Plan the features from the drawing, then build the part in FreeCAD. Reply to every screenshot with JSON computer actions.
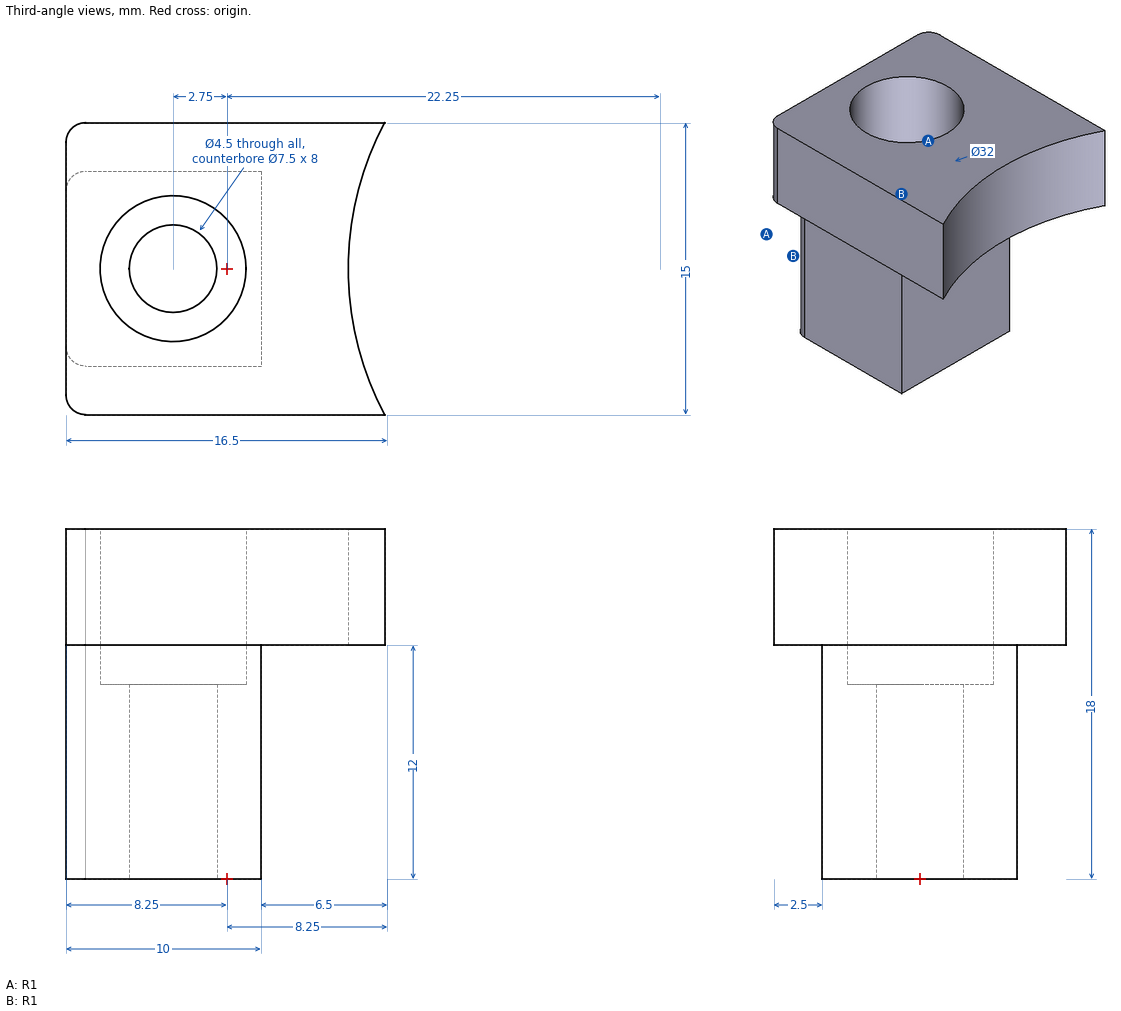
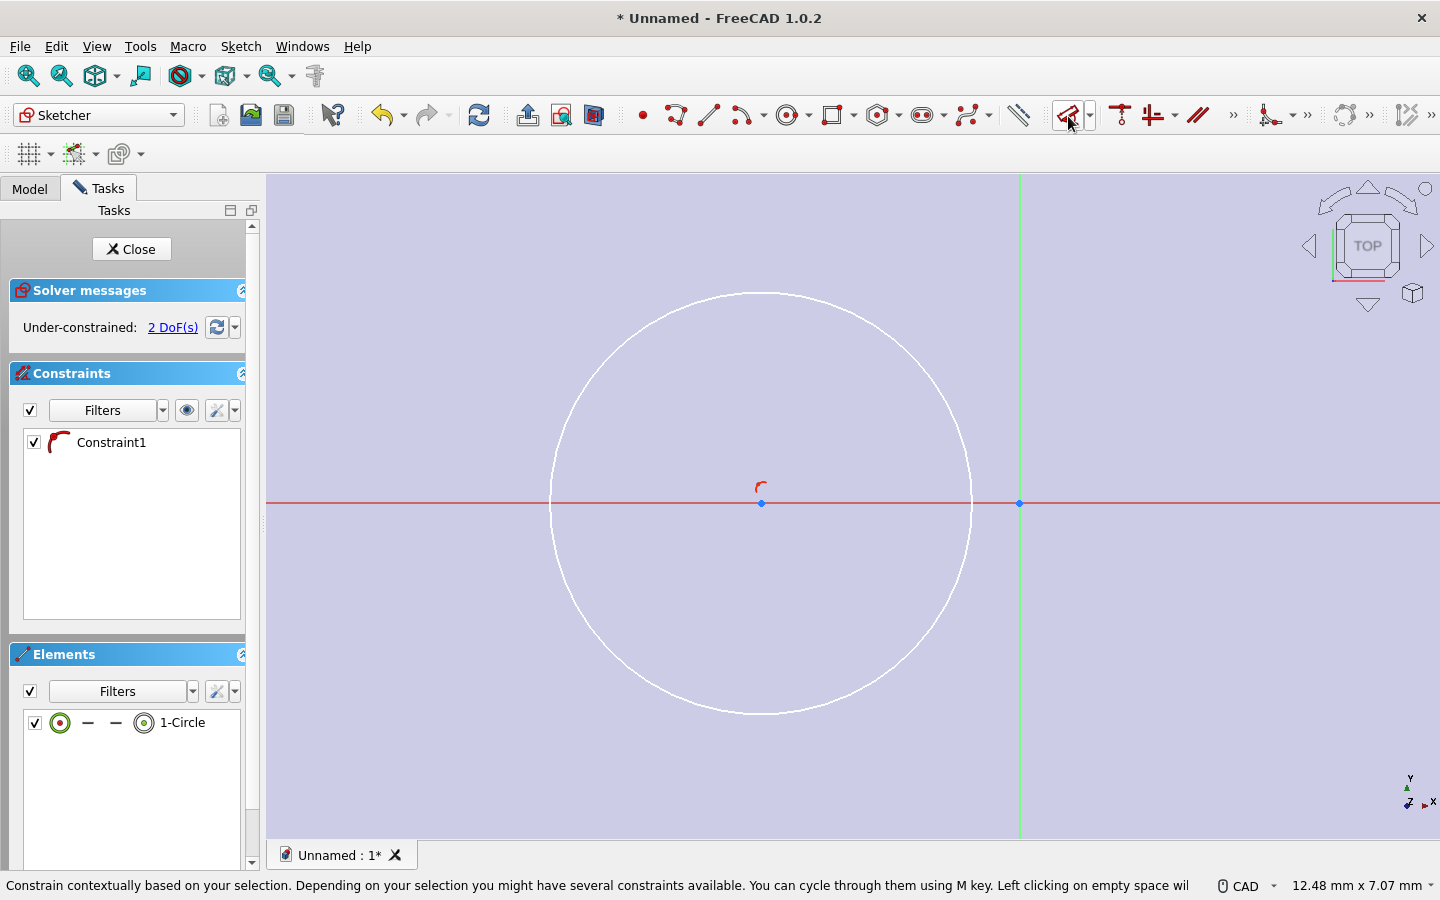
{"action": "left_click", "coordinate": [910, 354]}
{"action": "left_click", "coordinate": [933, 331]}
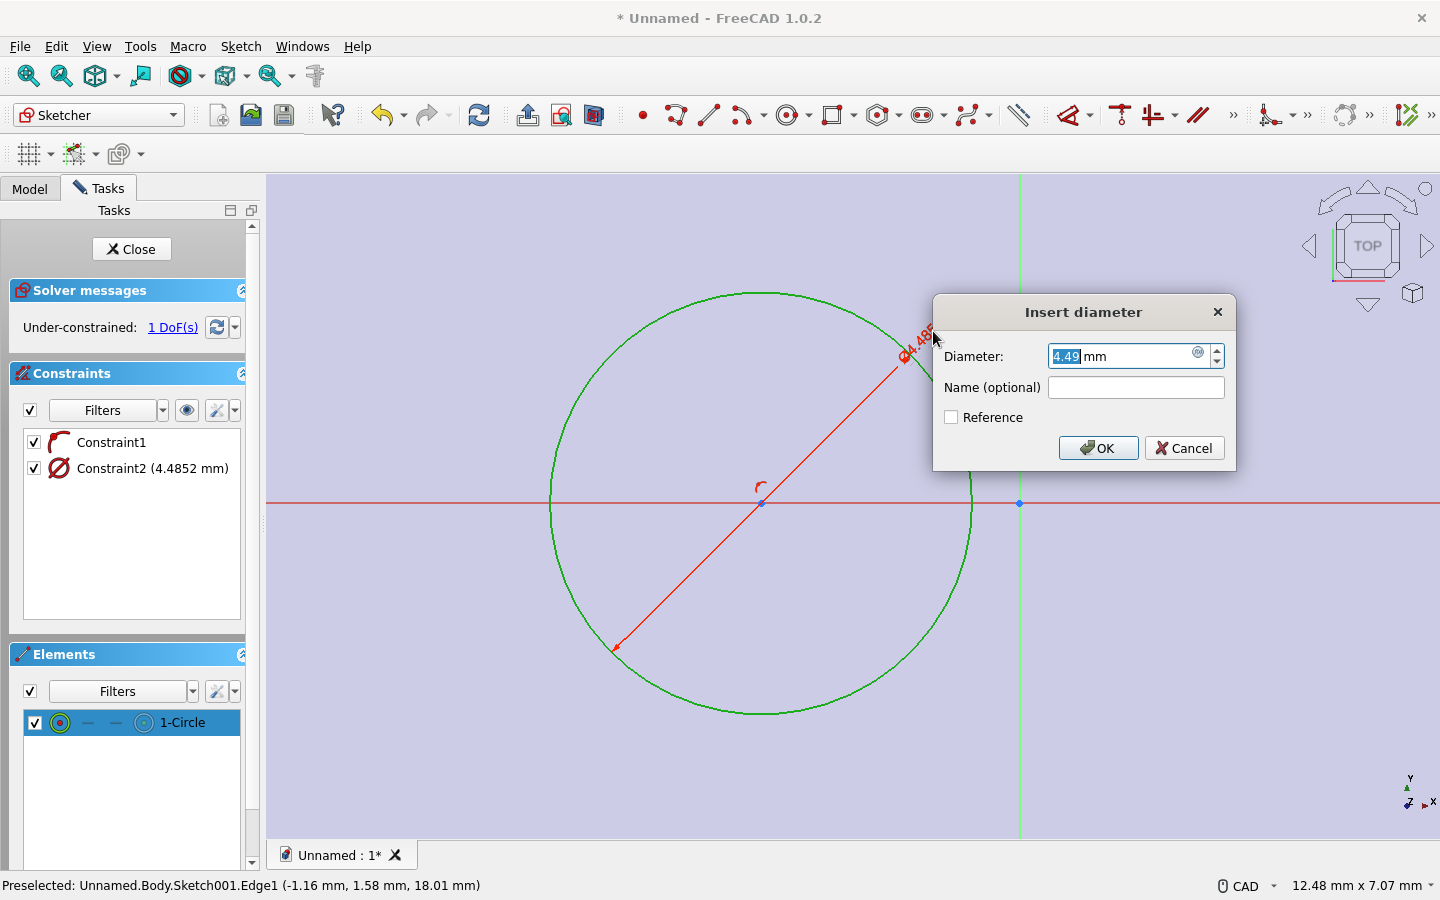
{"action": "type", "text": "4.5"}
{"action": "key", "text": "Return"}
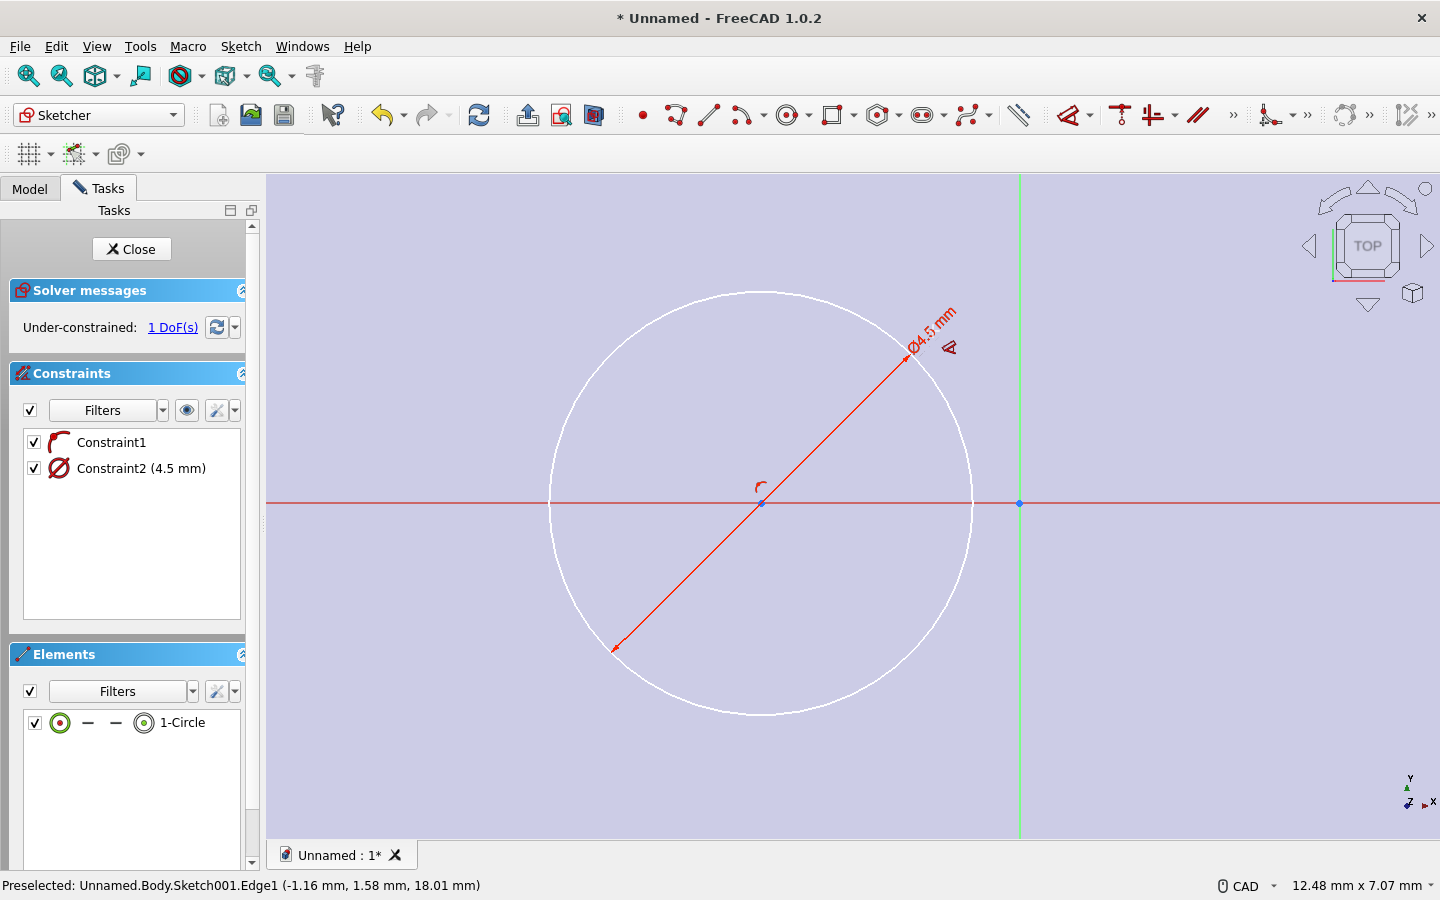
{"action": "left_click", "coordinate": [761, 503]}
{"action": "left_click", "coordinate": [890, 537]}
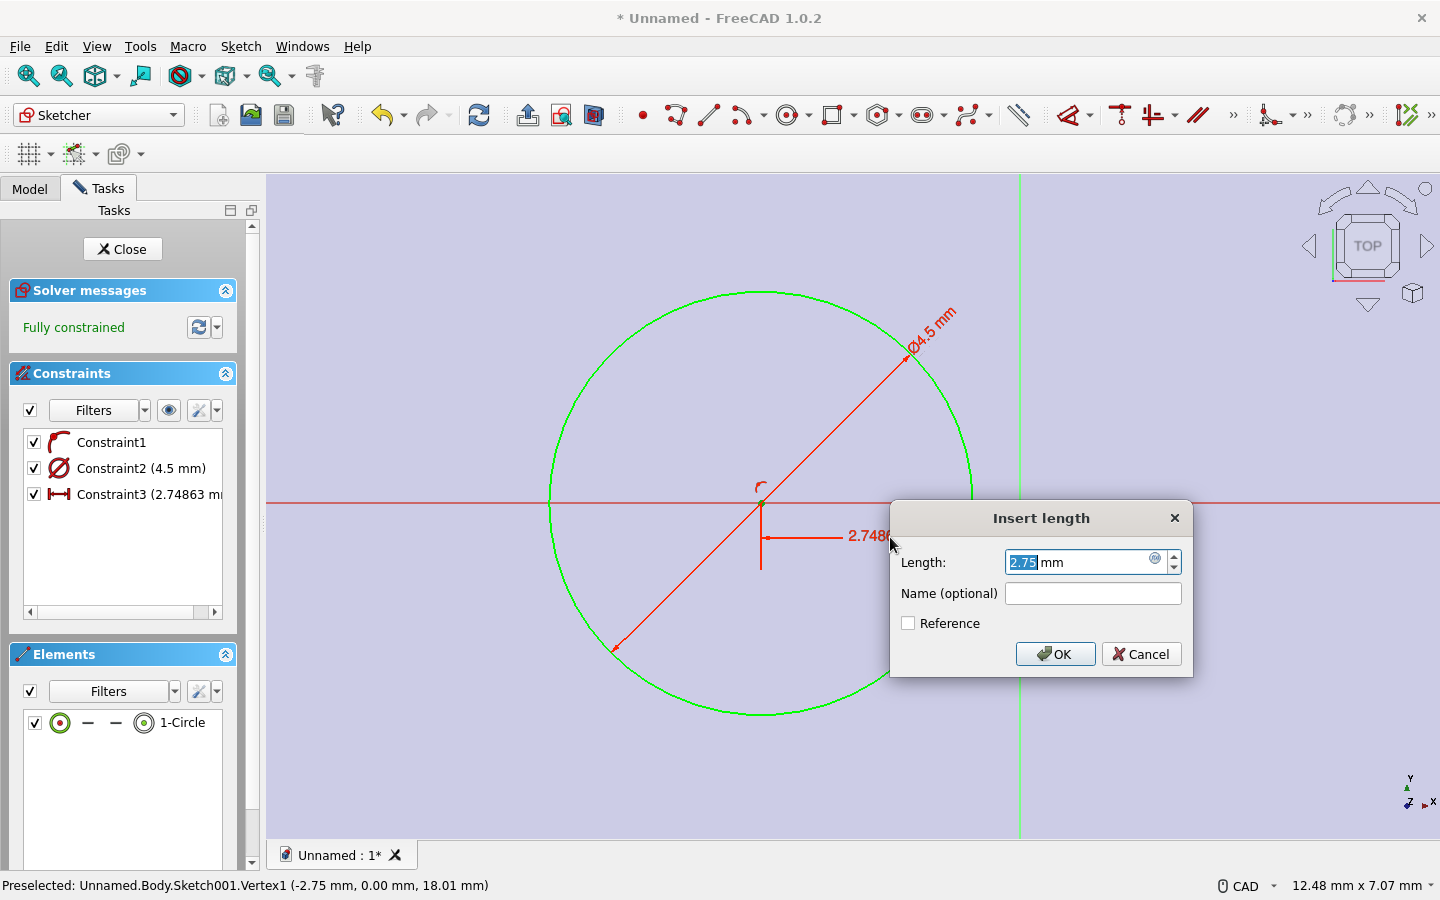
{"action": "type", "text": "2.75"}
{"action": "key", "text": "Return"}
{"action": "key", "text": "Escape"}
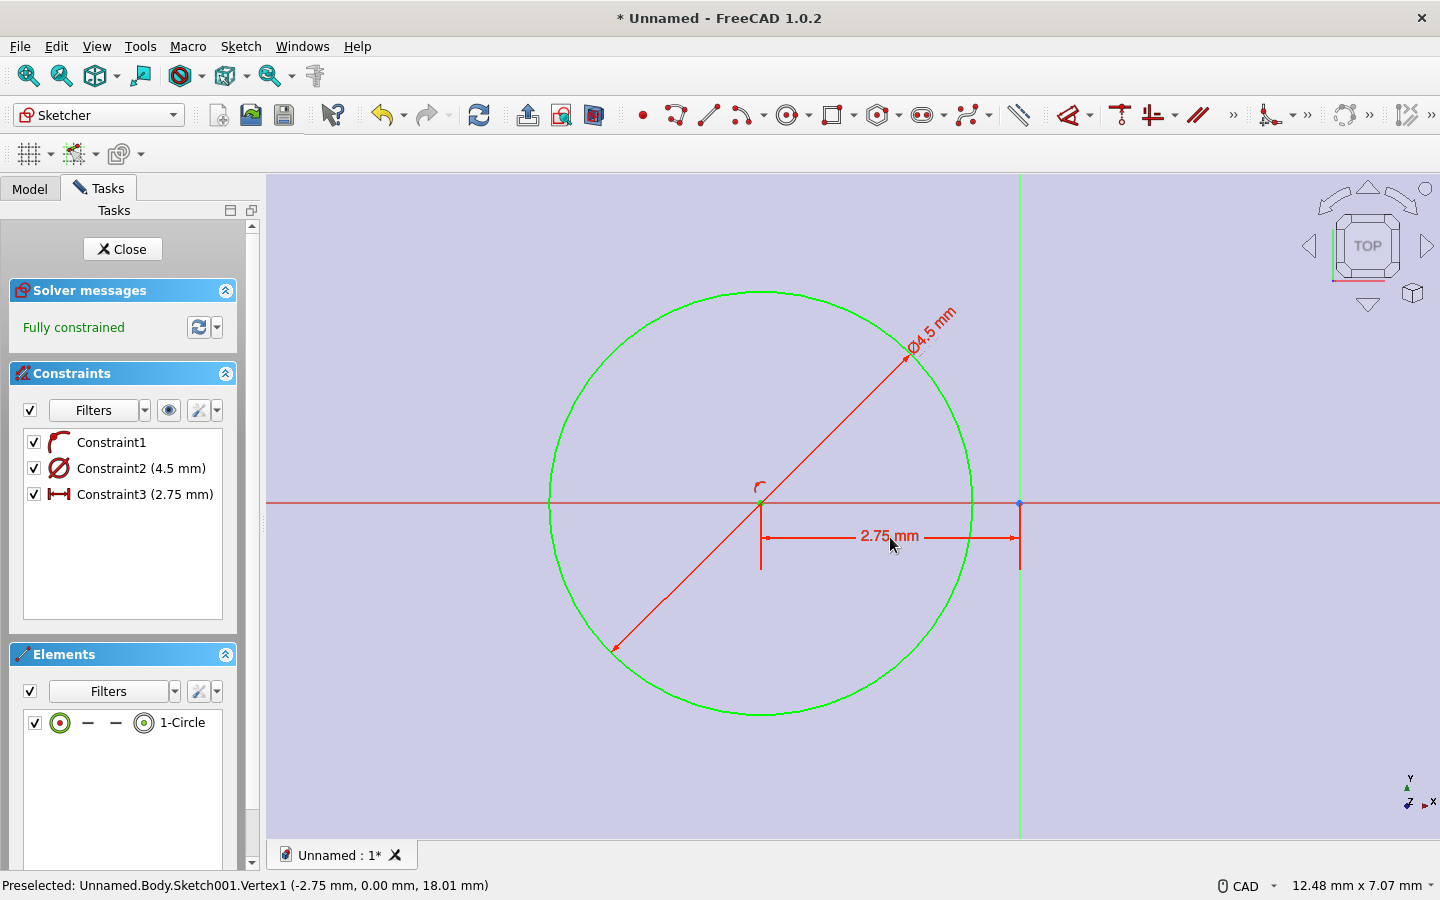
{"action": "left_click", "coordinate": [123, 249]}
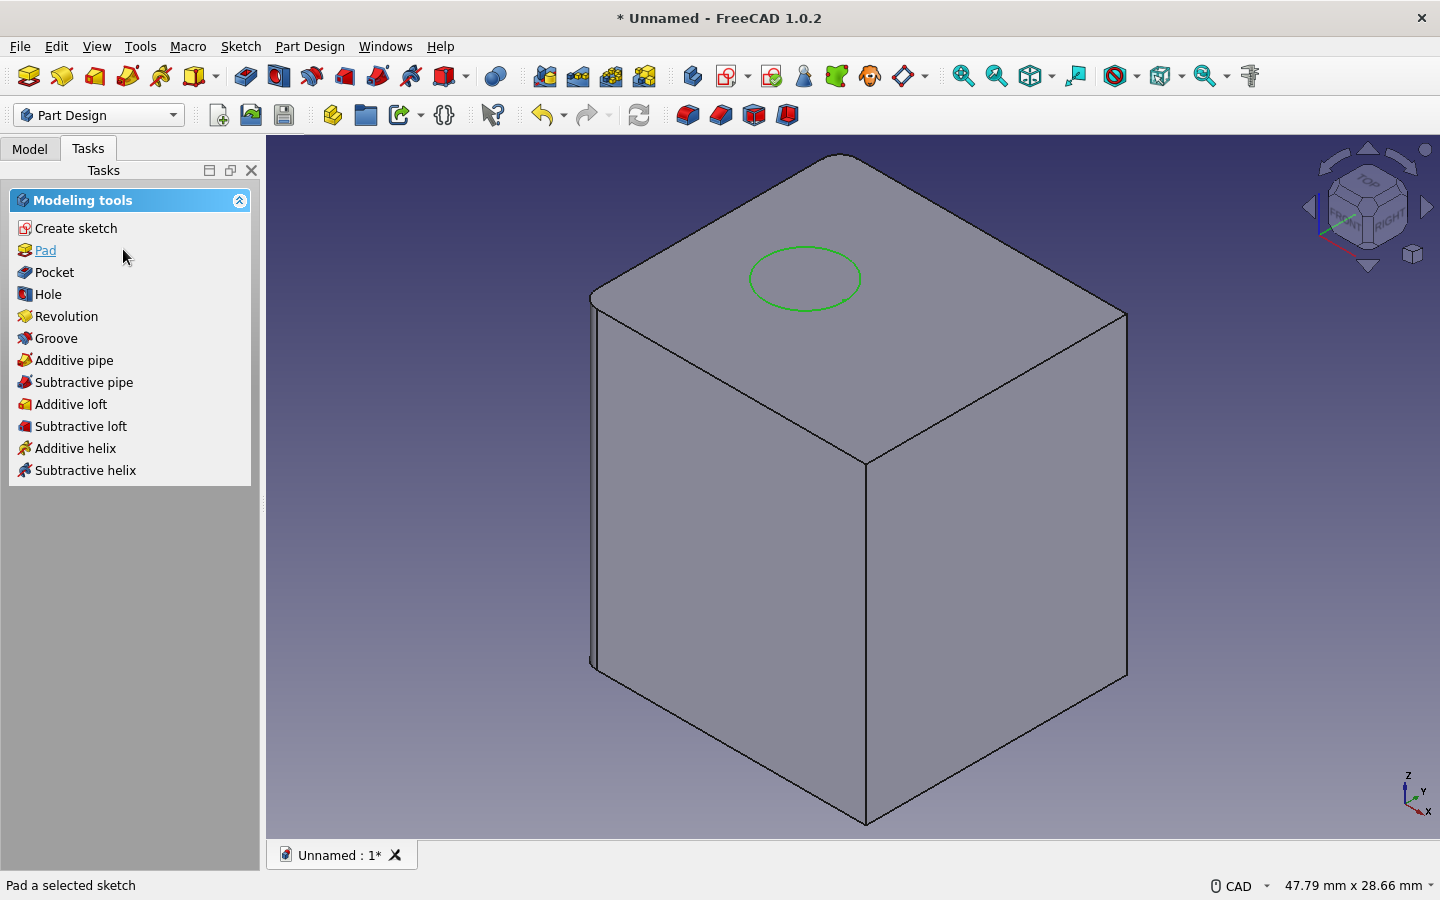
{"action": "left_click", "coordinate": [279, 76]}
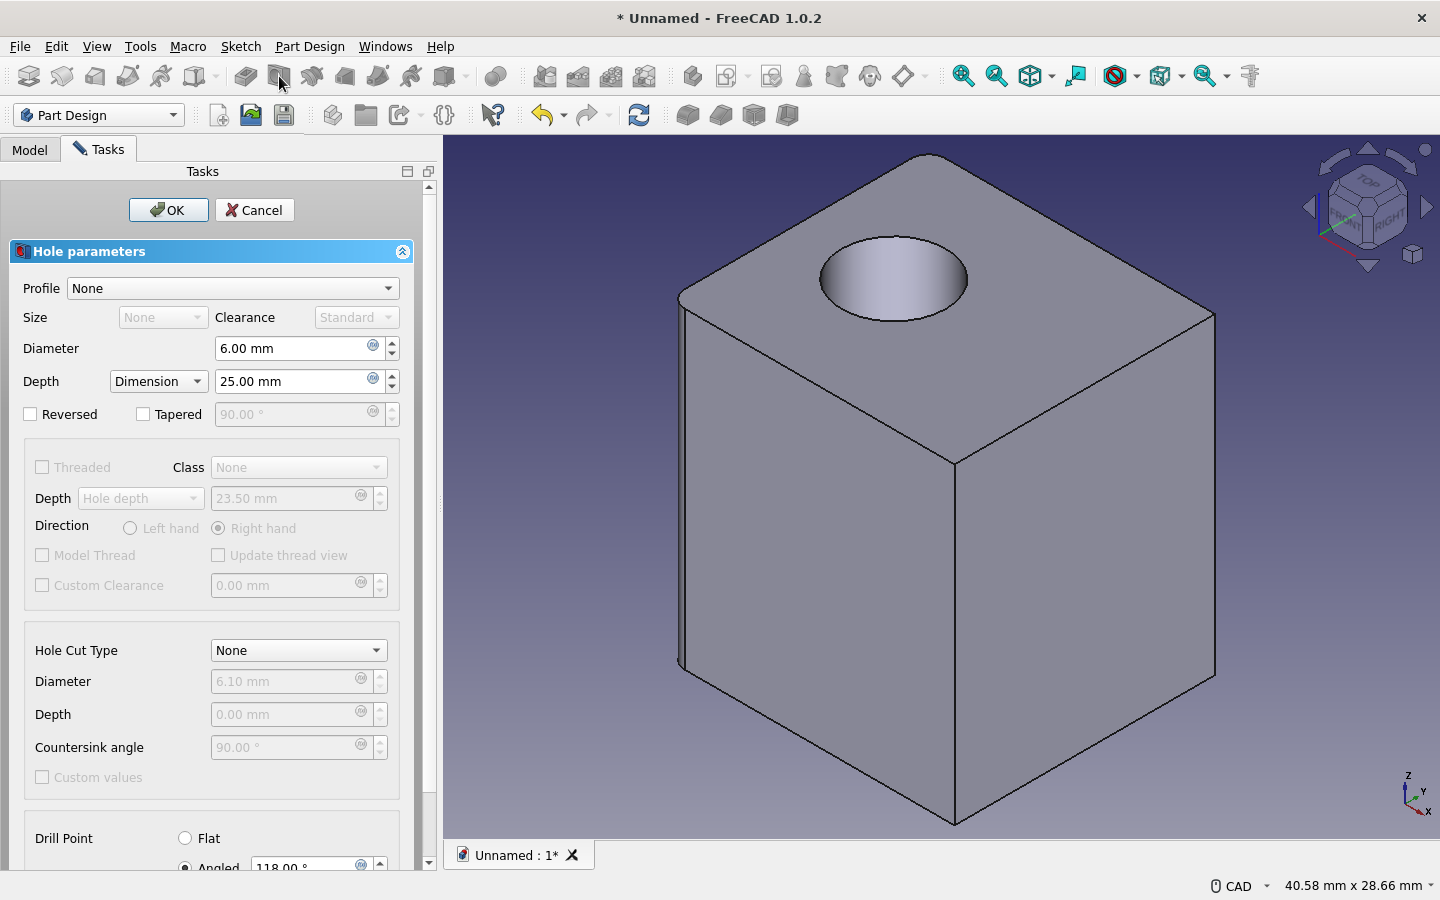
{"action": "triple_click", "coordinate": [300, 348]}